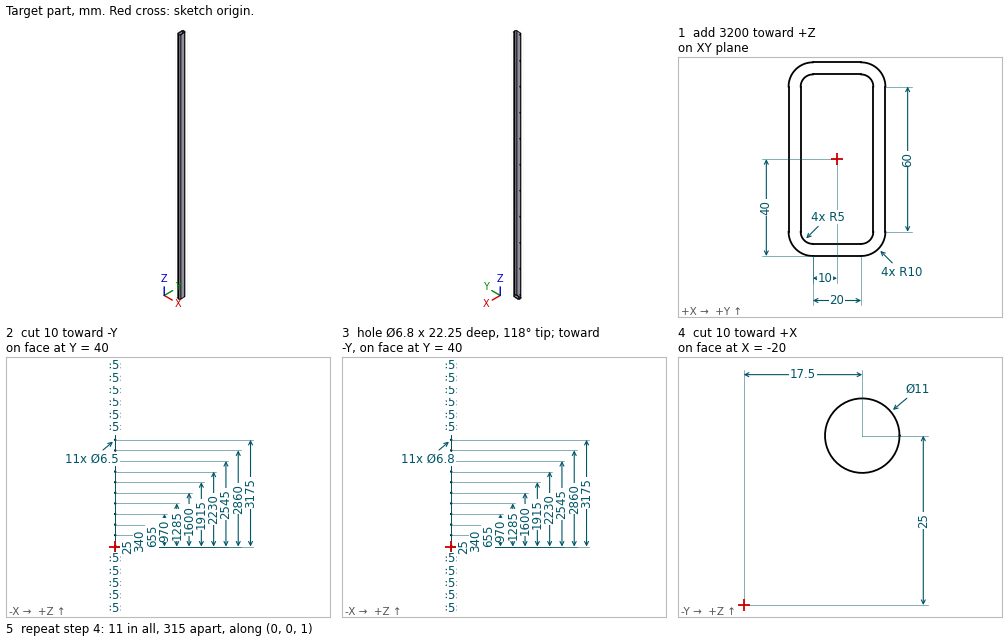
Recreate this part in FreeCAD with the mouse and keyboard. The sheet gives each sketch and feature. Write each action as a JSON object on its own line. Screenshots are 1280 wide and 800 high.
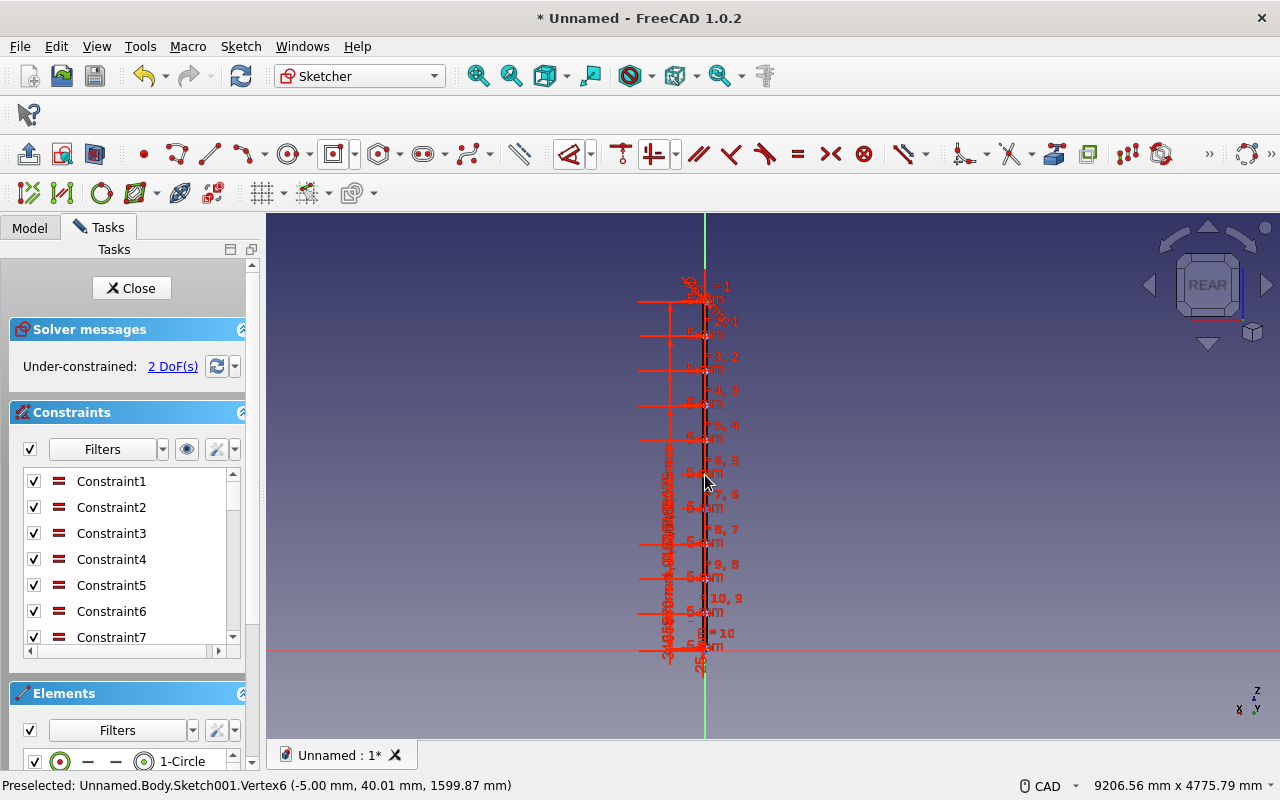
{"action": "key", "text": "i"}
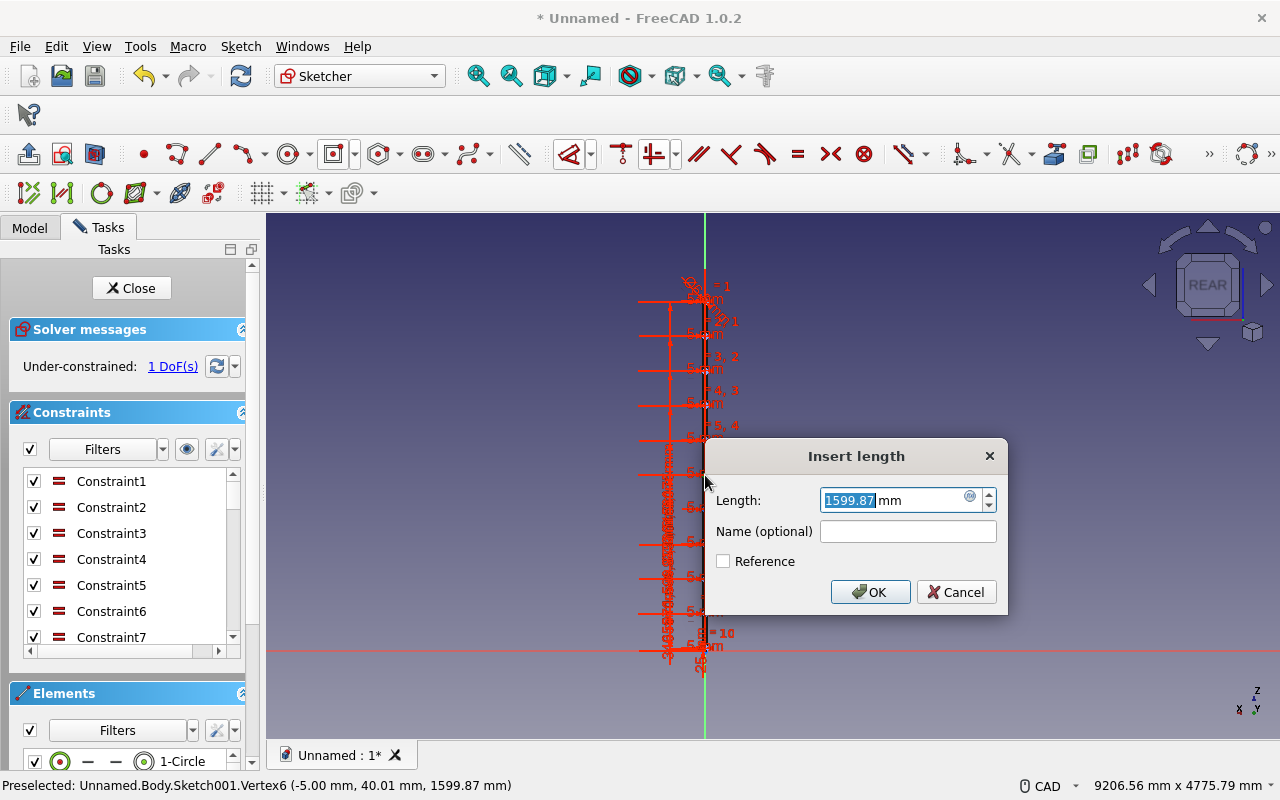
{"action": "type", "text": "1600"}
{"action": "key", "text": "Return"}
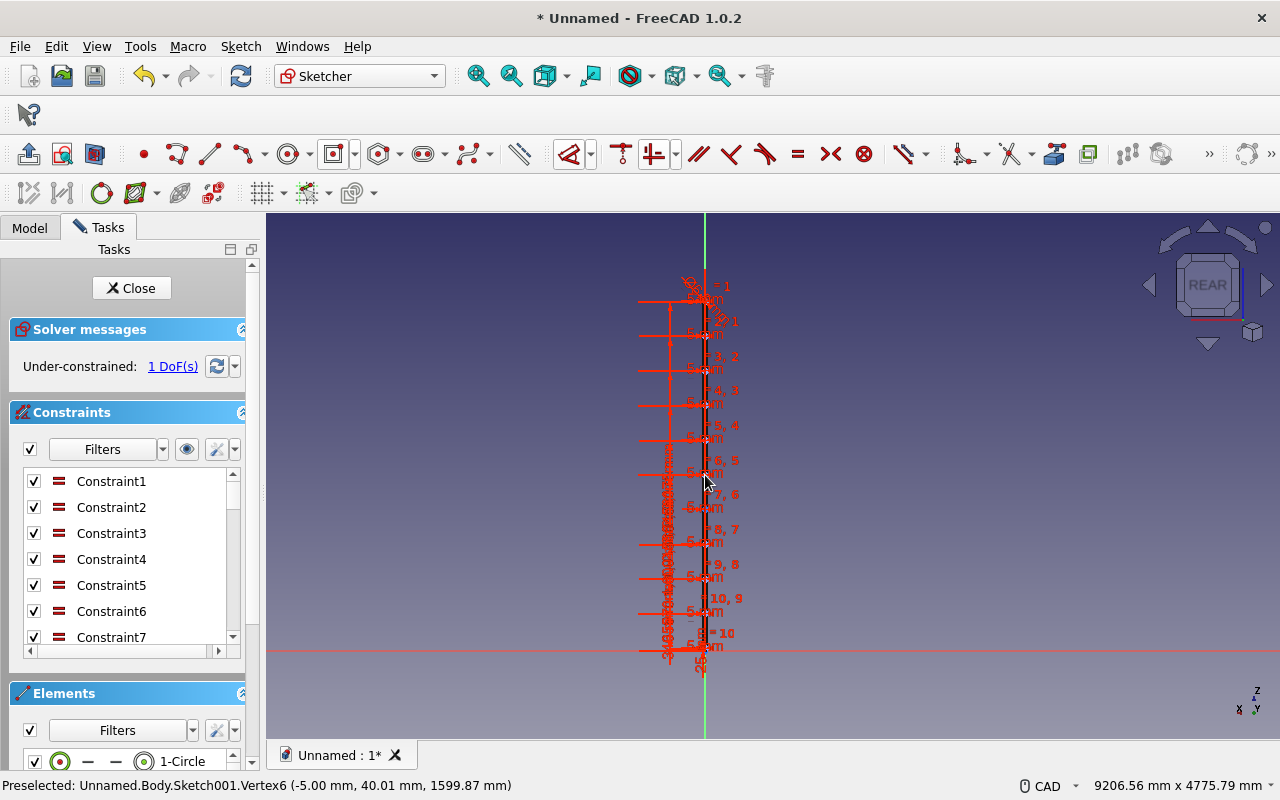
{"action": "left_click", "coordinate": [705, 510]}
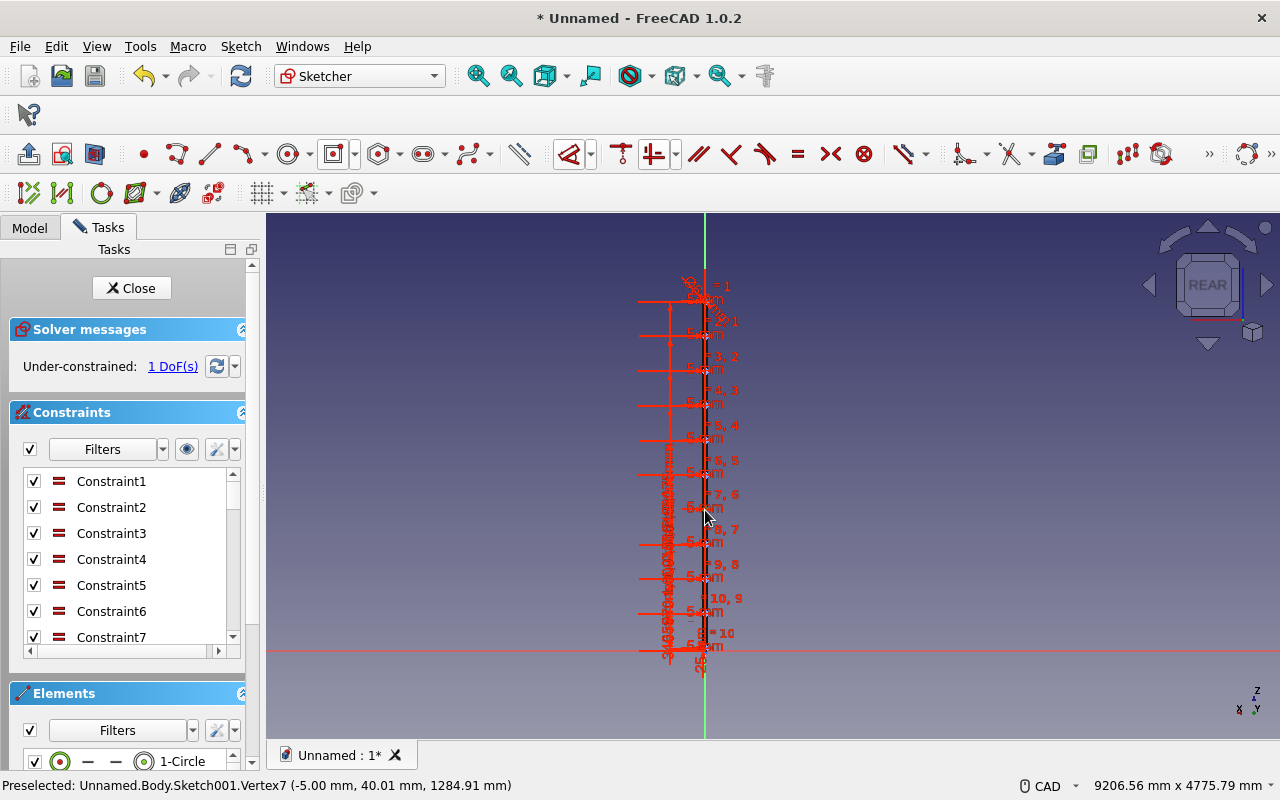
{"action": "left_click", "coordinate": [590, 154]}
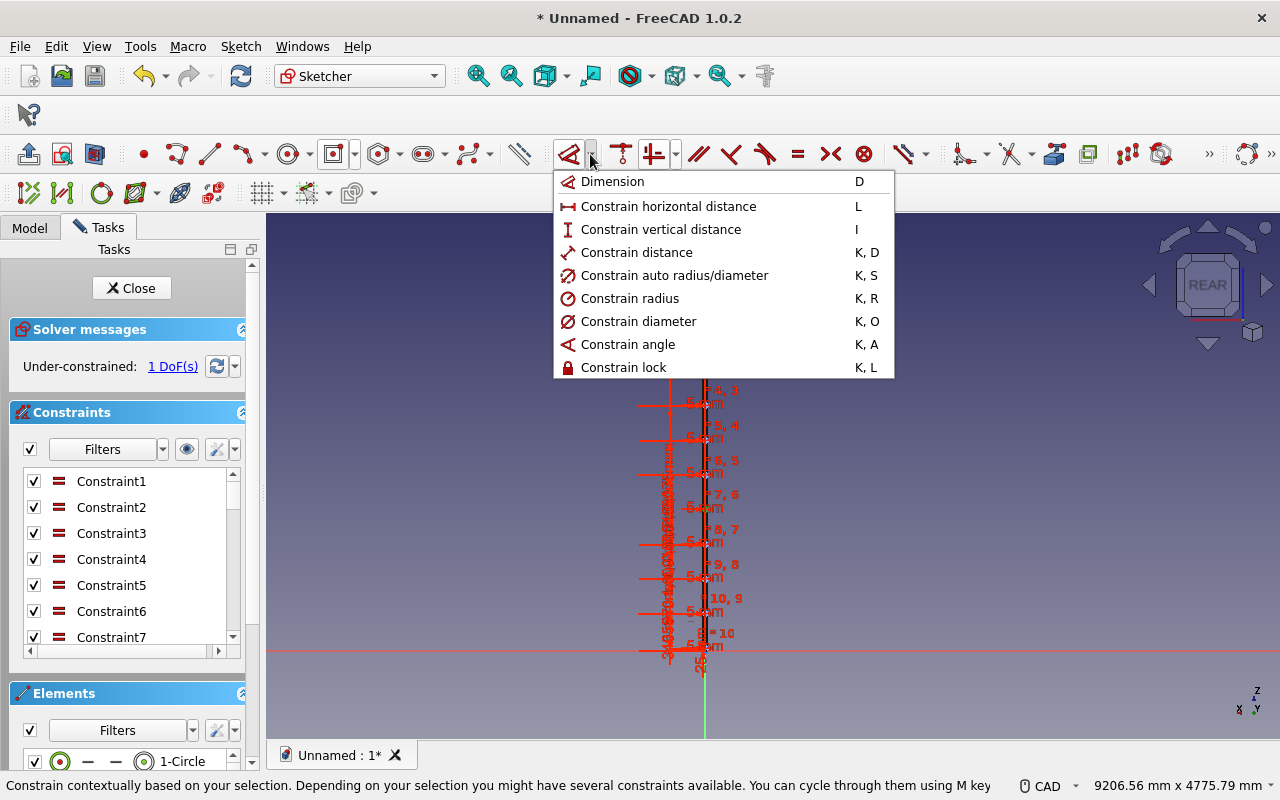
{"action": "left_click", "coordinate": [724, 230]}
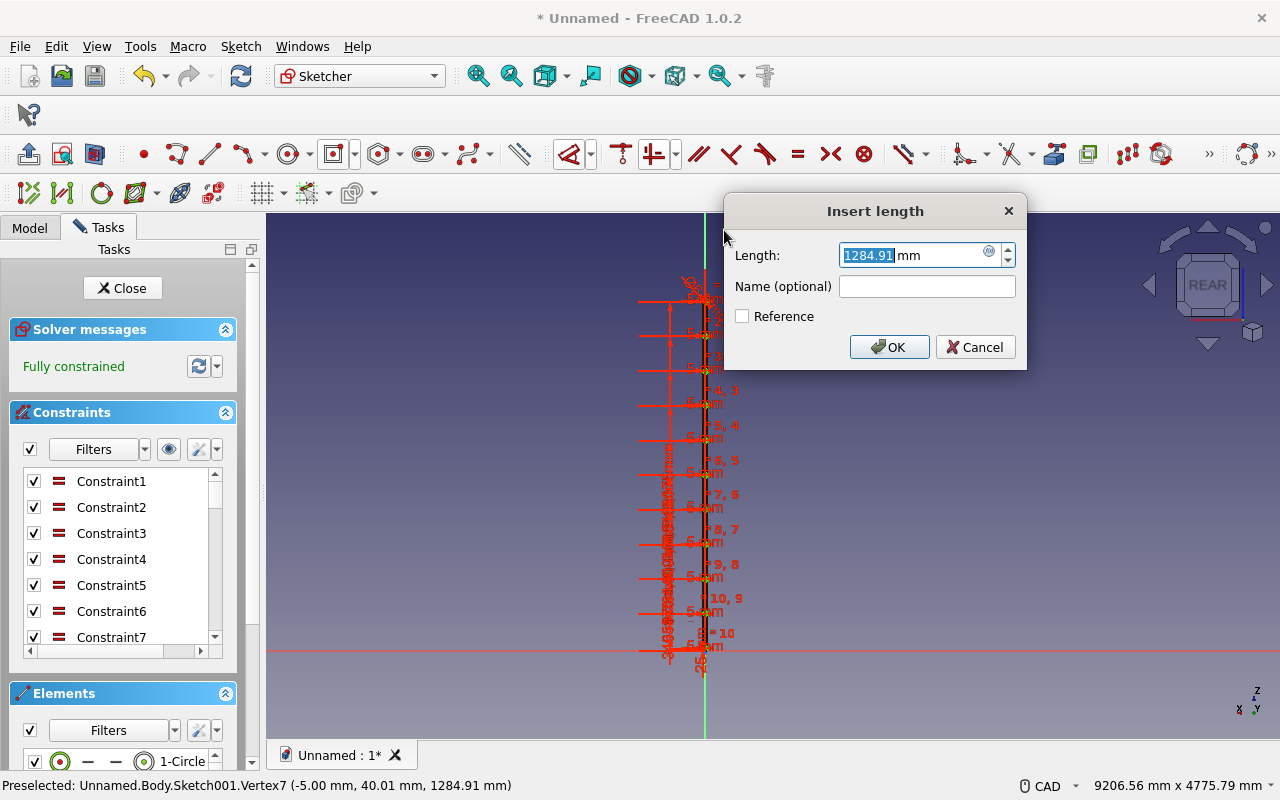
{"action": "type", "text": "1285"}
{"action": "key", "text": "Return"}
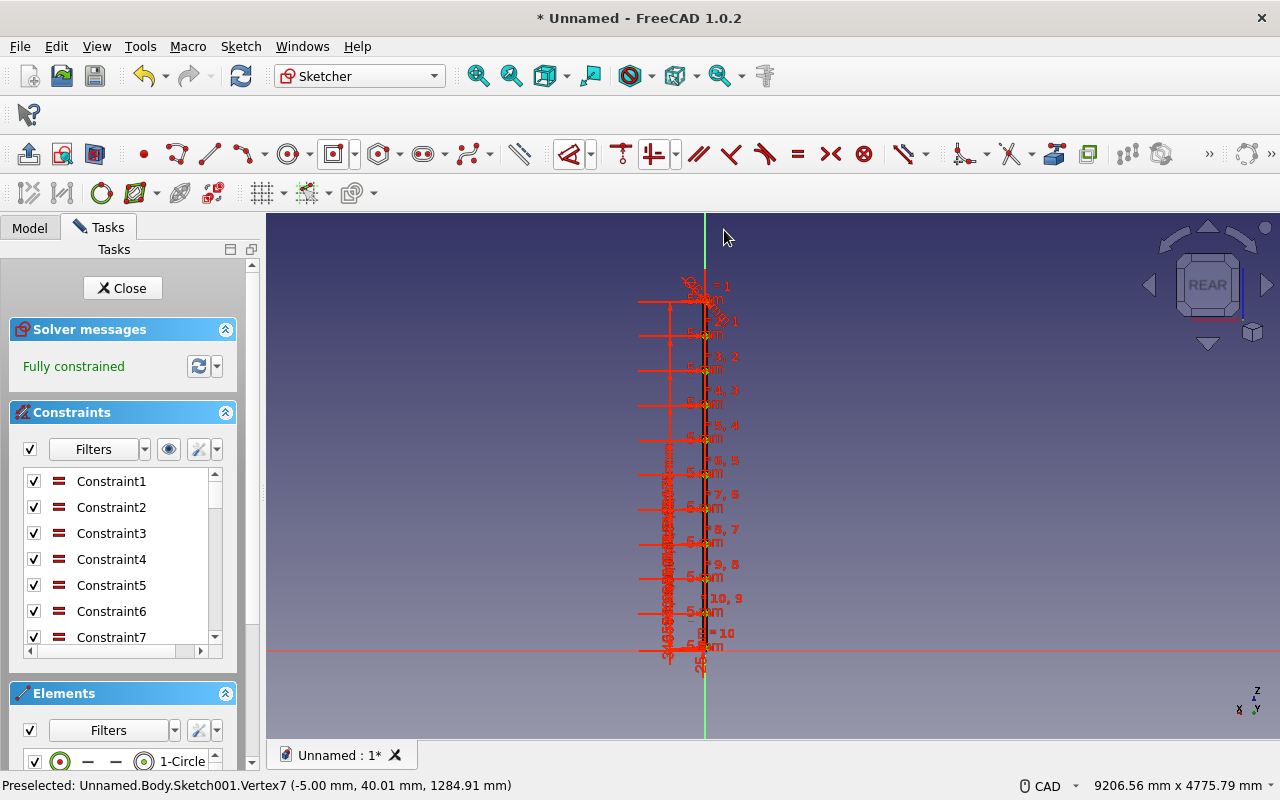
{"action": "left_click", "coordinate": [123, 288]}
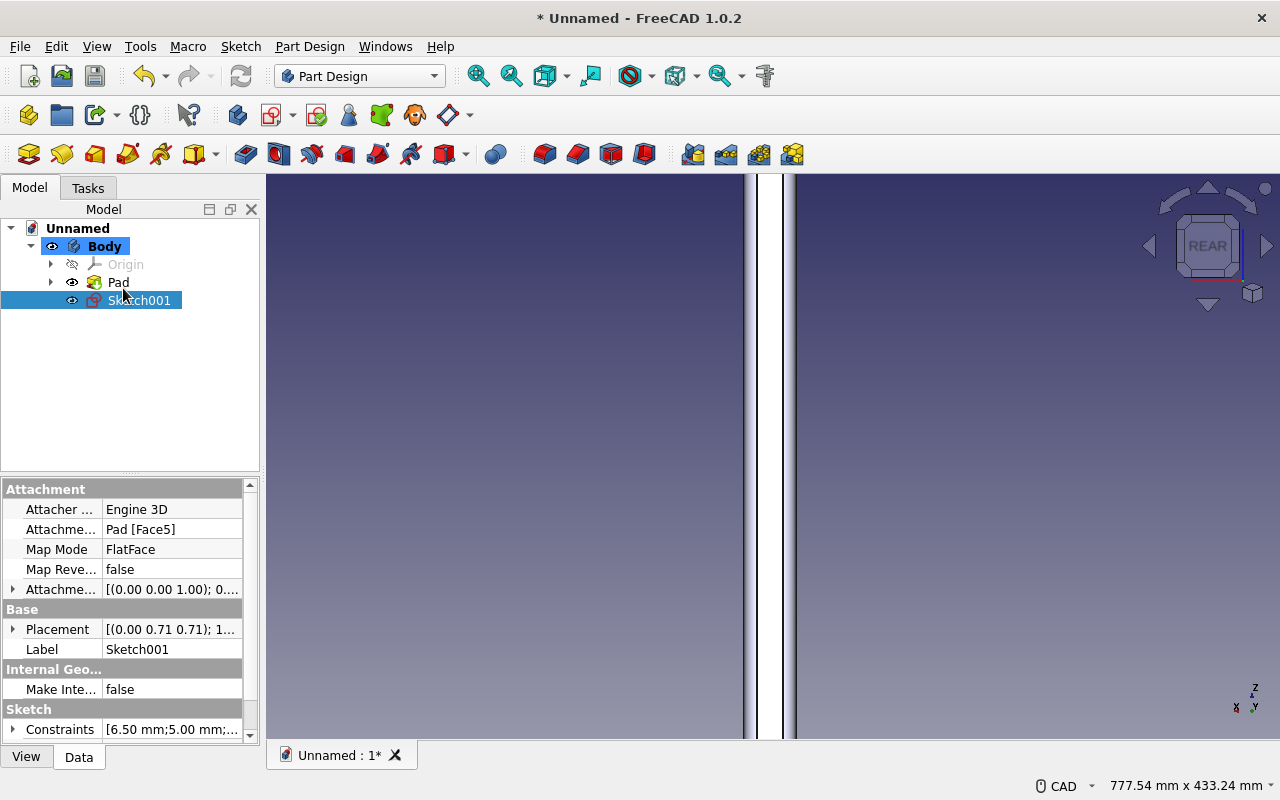
{"action": "left_click", "coordinate": [246, 154]}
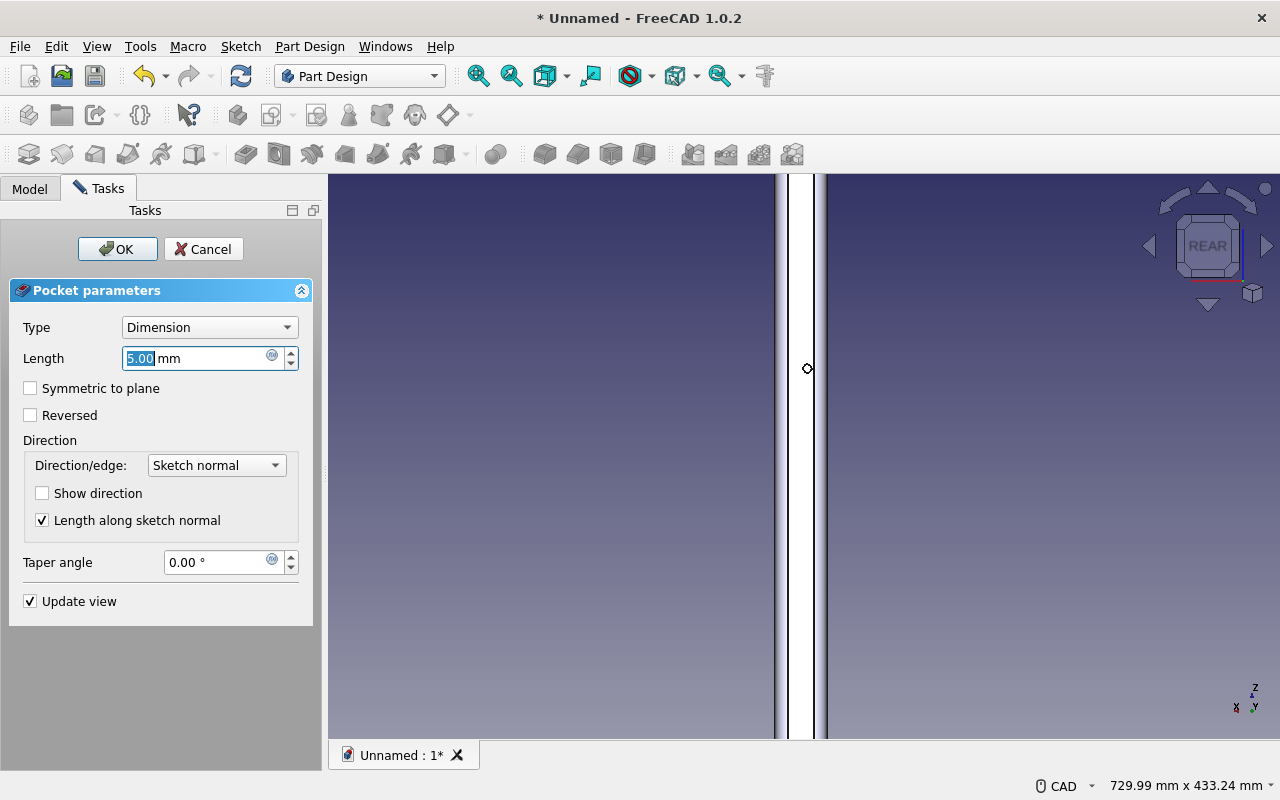
{"action": "type", "text": "10"}
{"action": "key", "text": "Tab"}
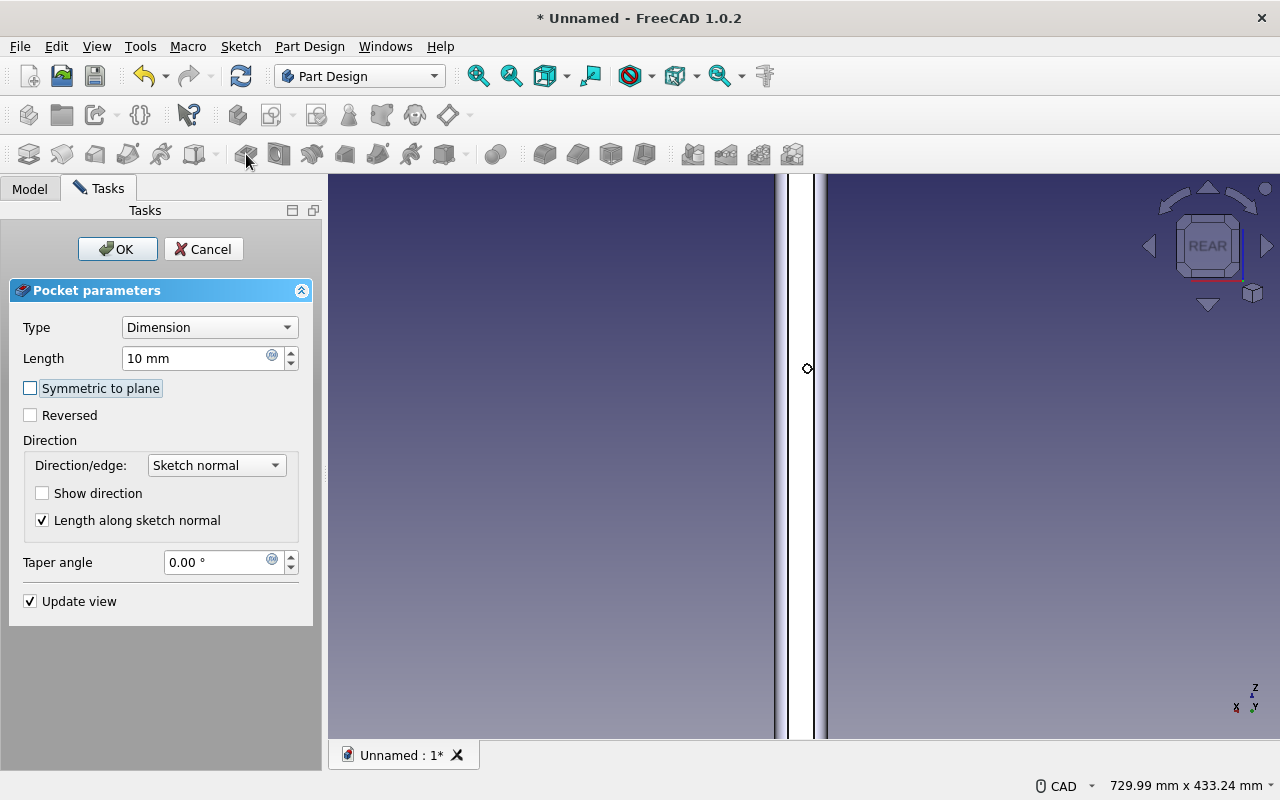
{"action": "left_click", "coordinate": [118, 249]}